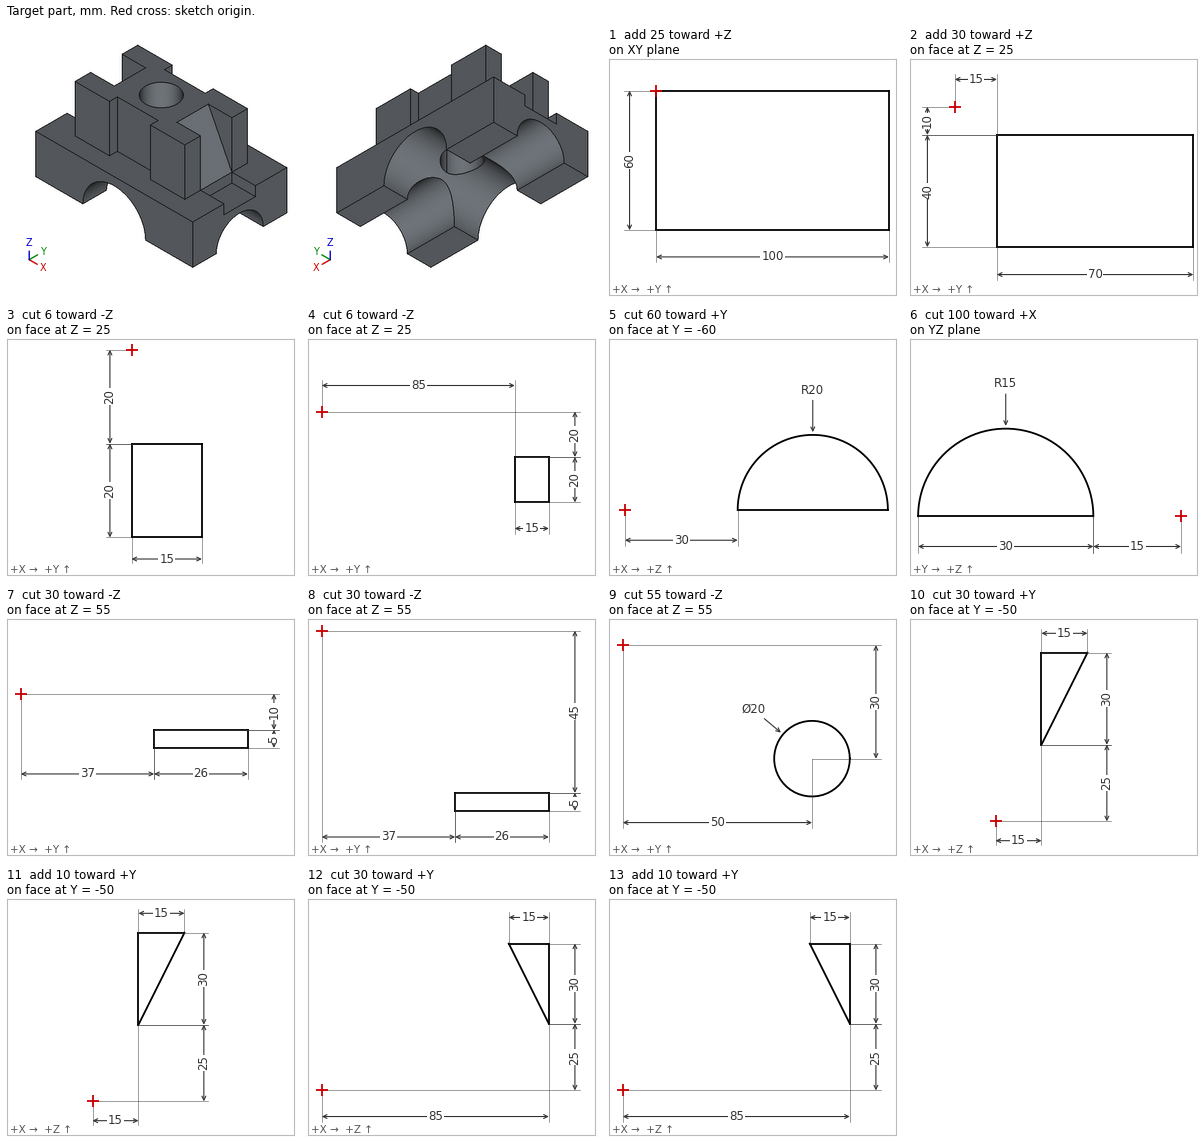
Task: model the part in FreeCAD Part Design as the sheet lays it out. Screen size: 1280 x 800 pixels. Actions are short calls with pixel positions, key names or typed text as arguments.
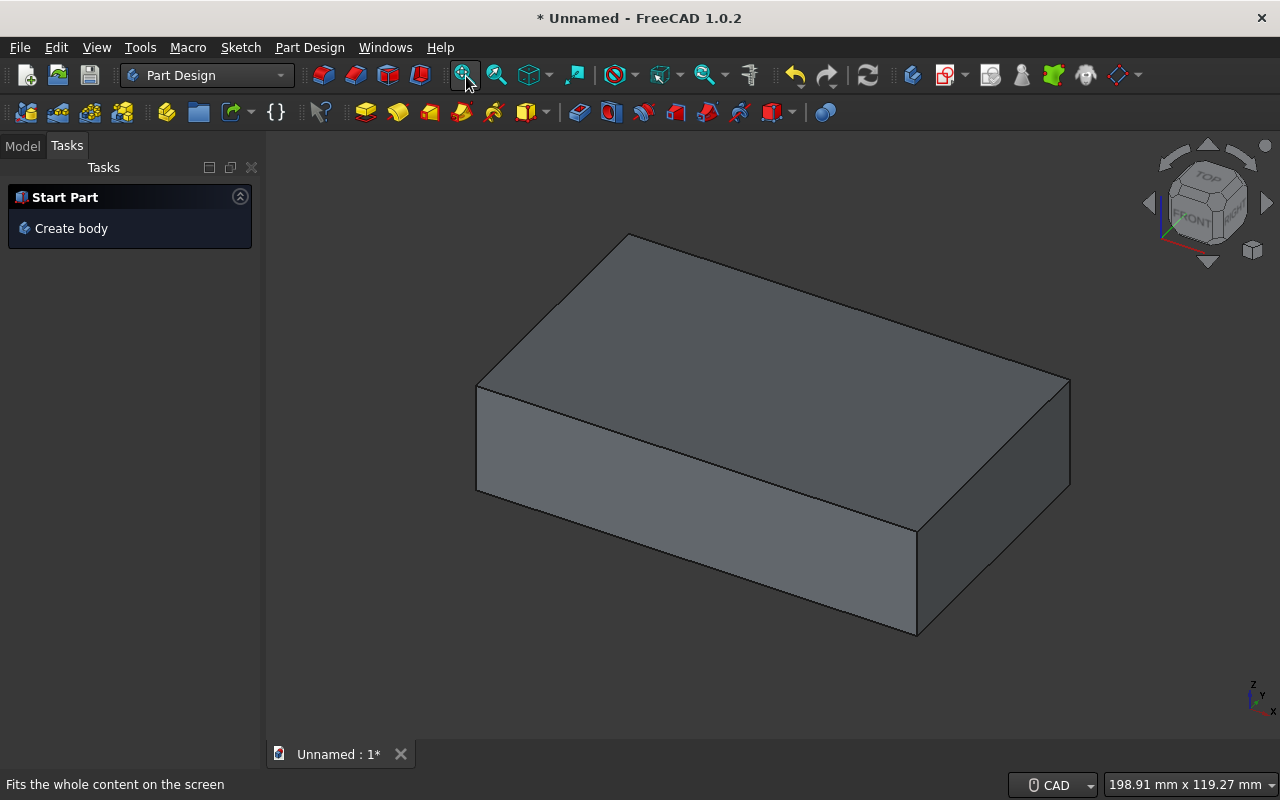
click(836, 403)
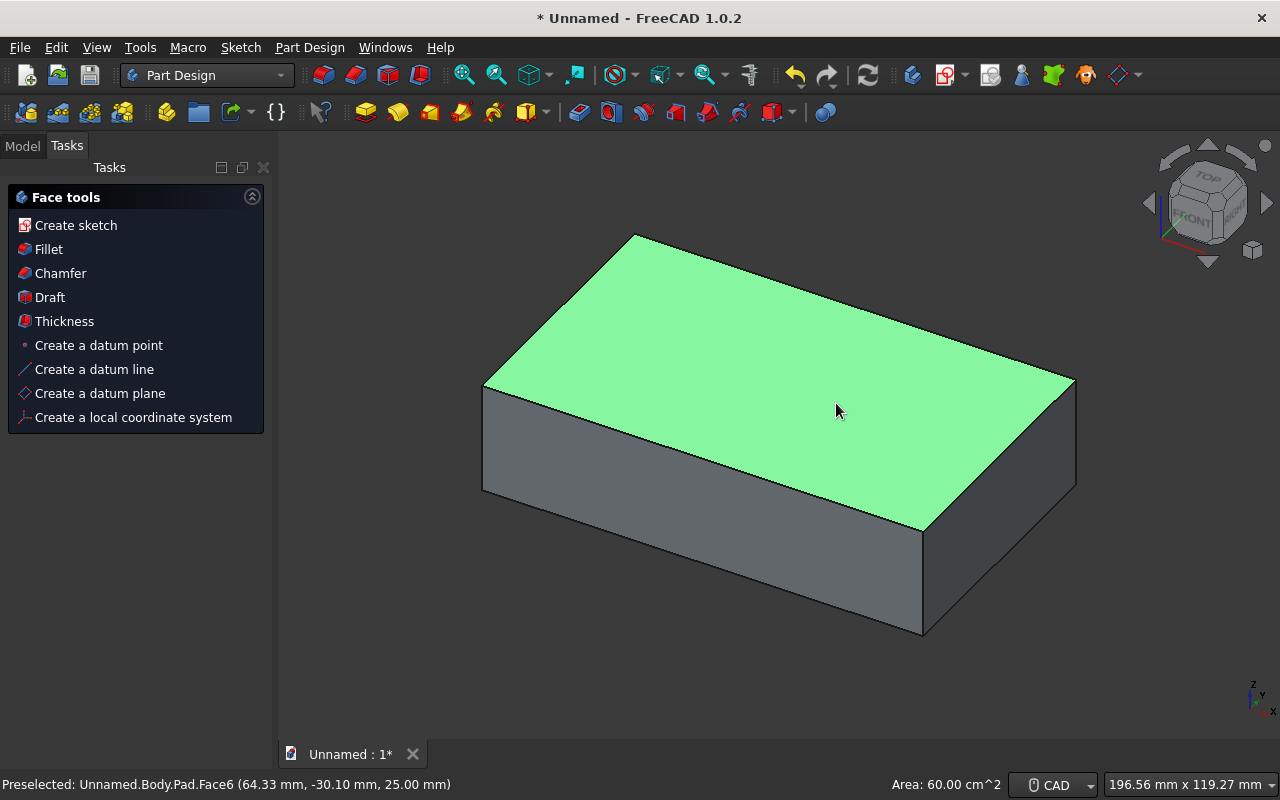
click(946, 76)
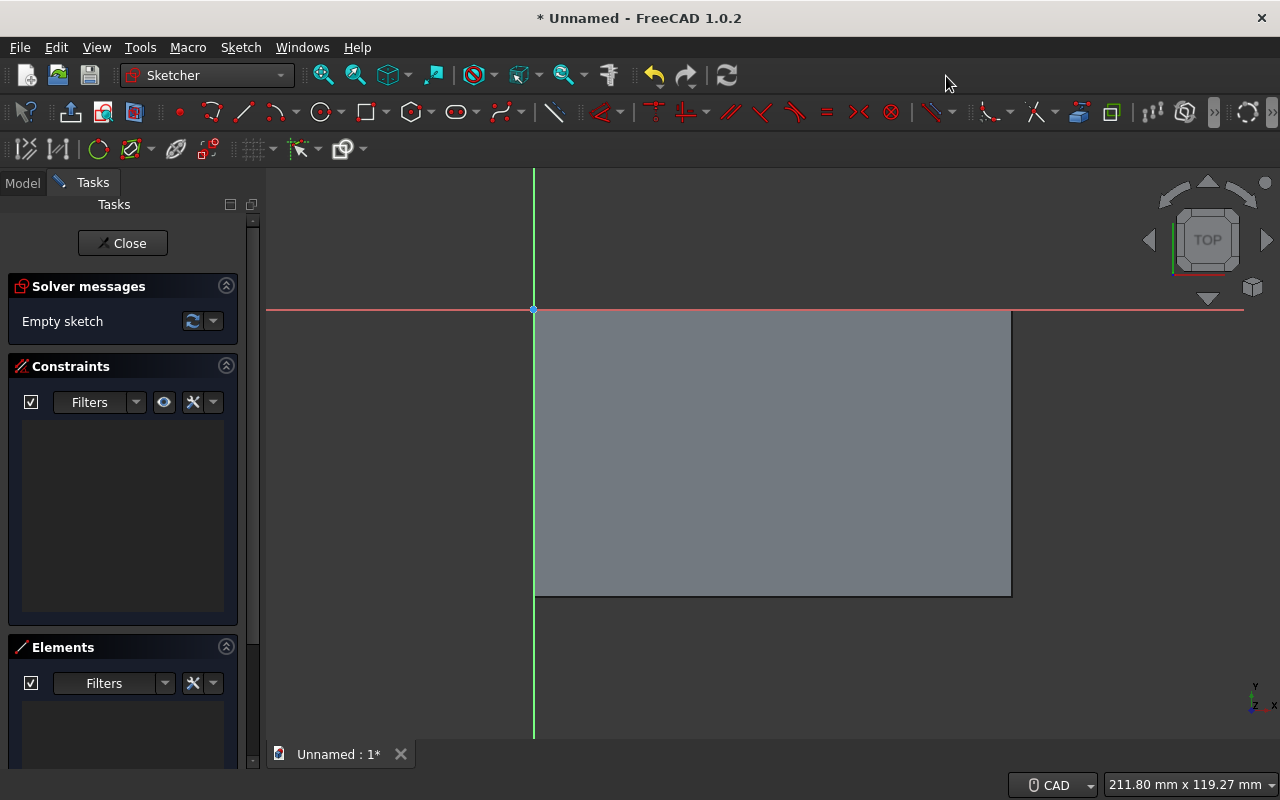
scroll(803, 381, up, 2)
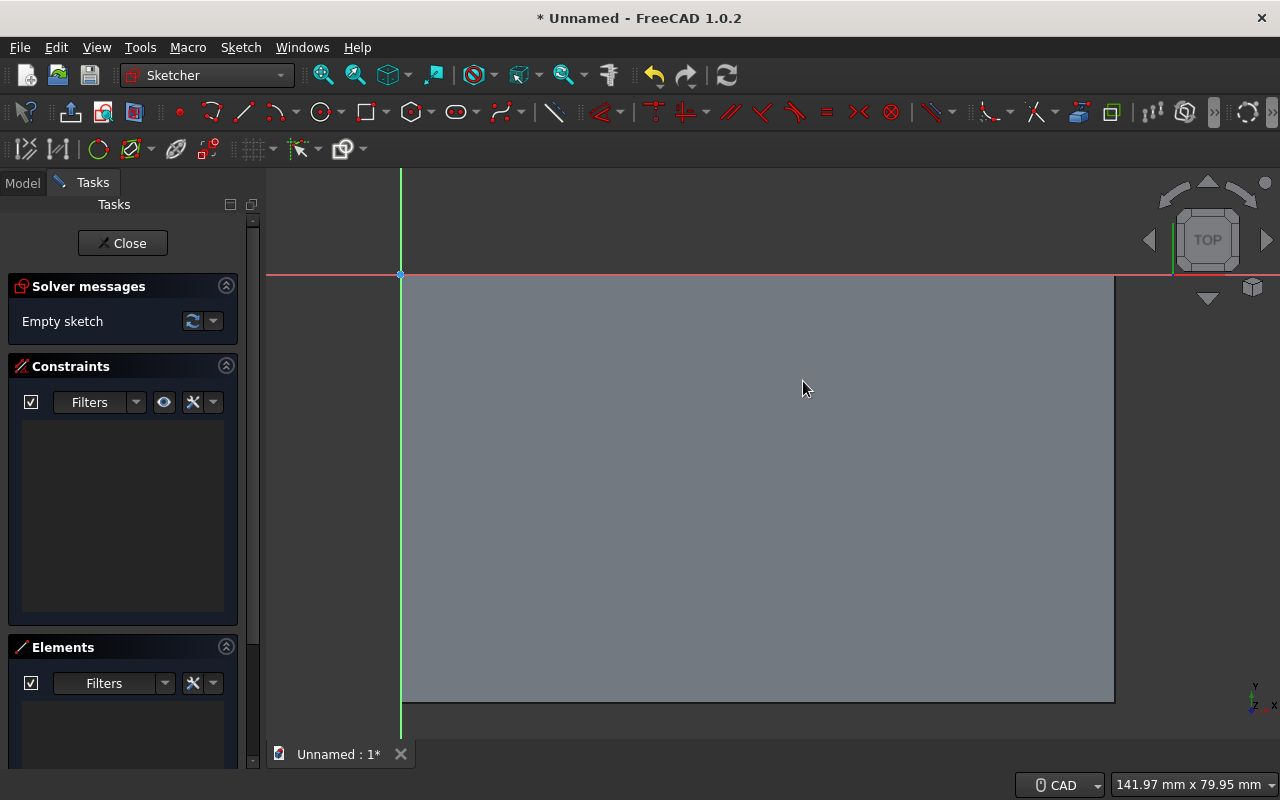
click(366, 112)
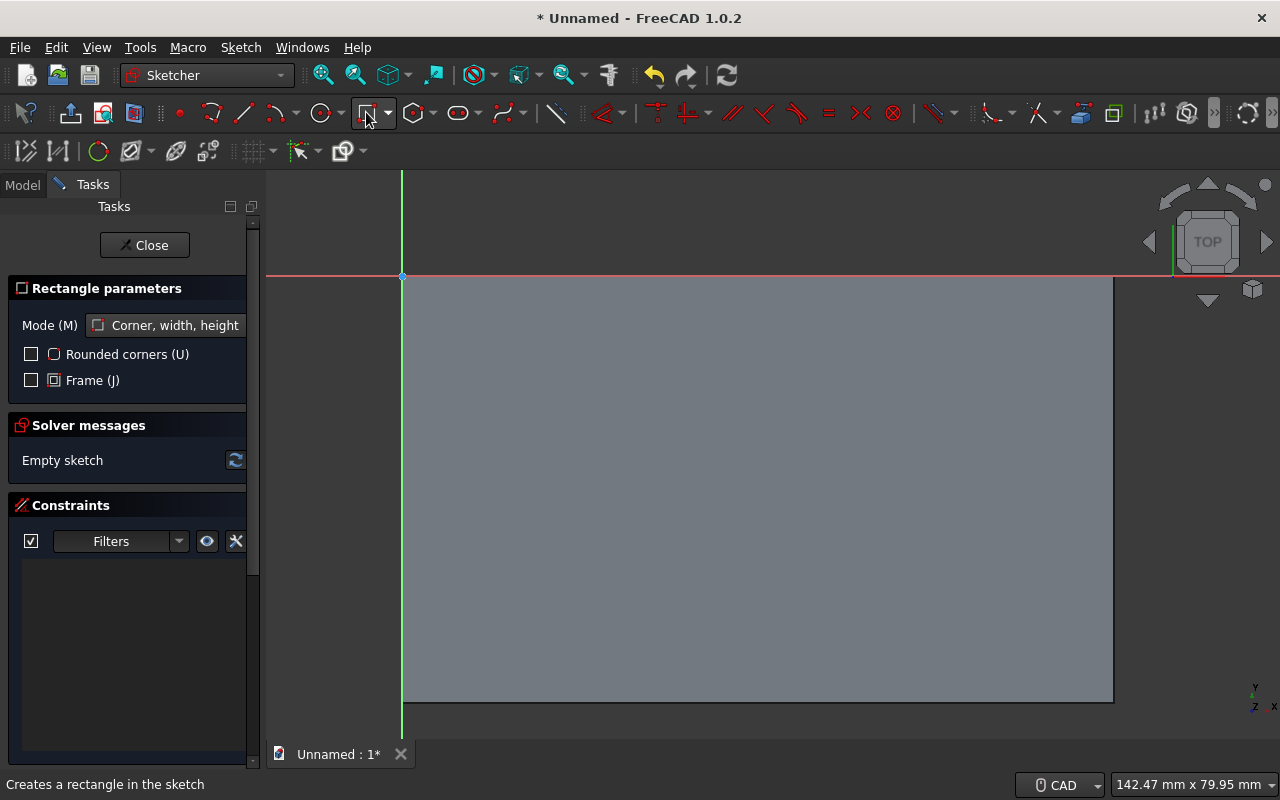
click(509, 348)
click(1007, 632)
key(Escape)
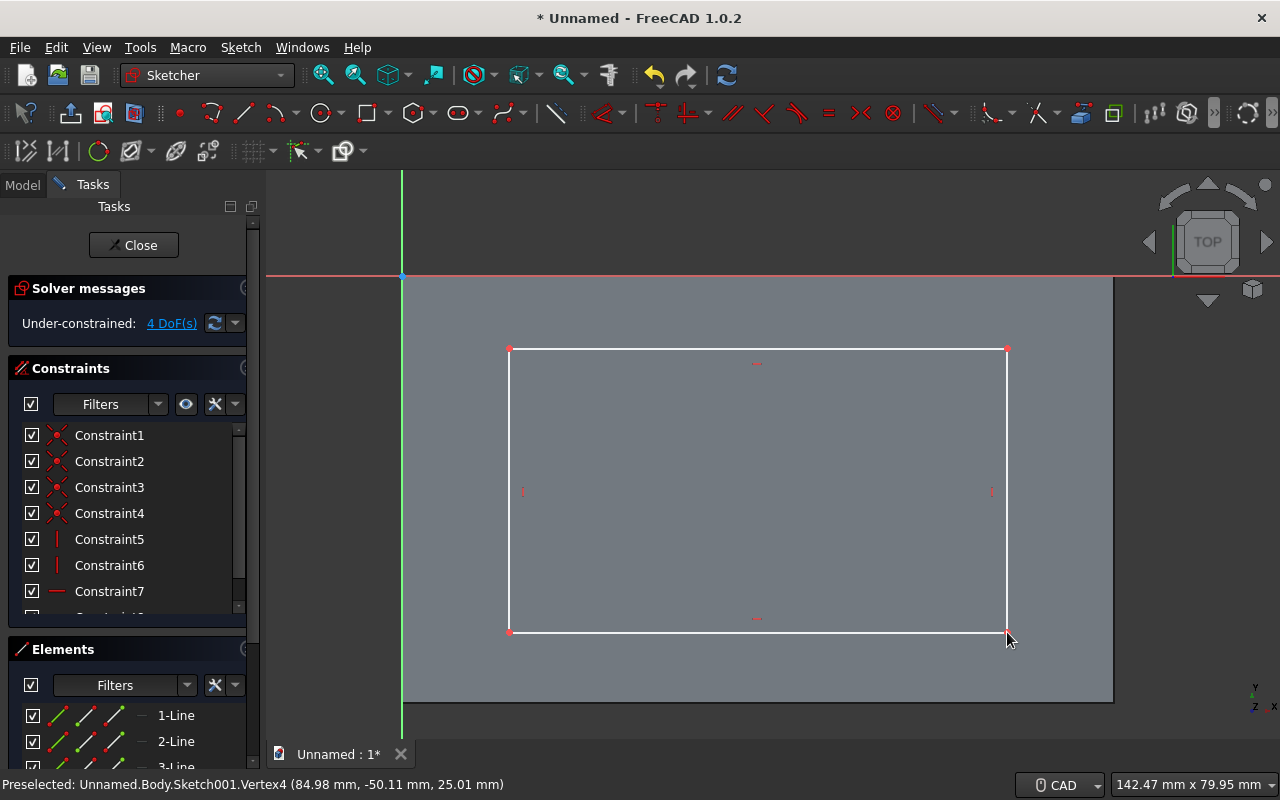
key(d)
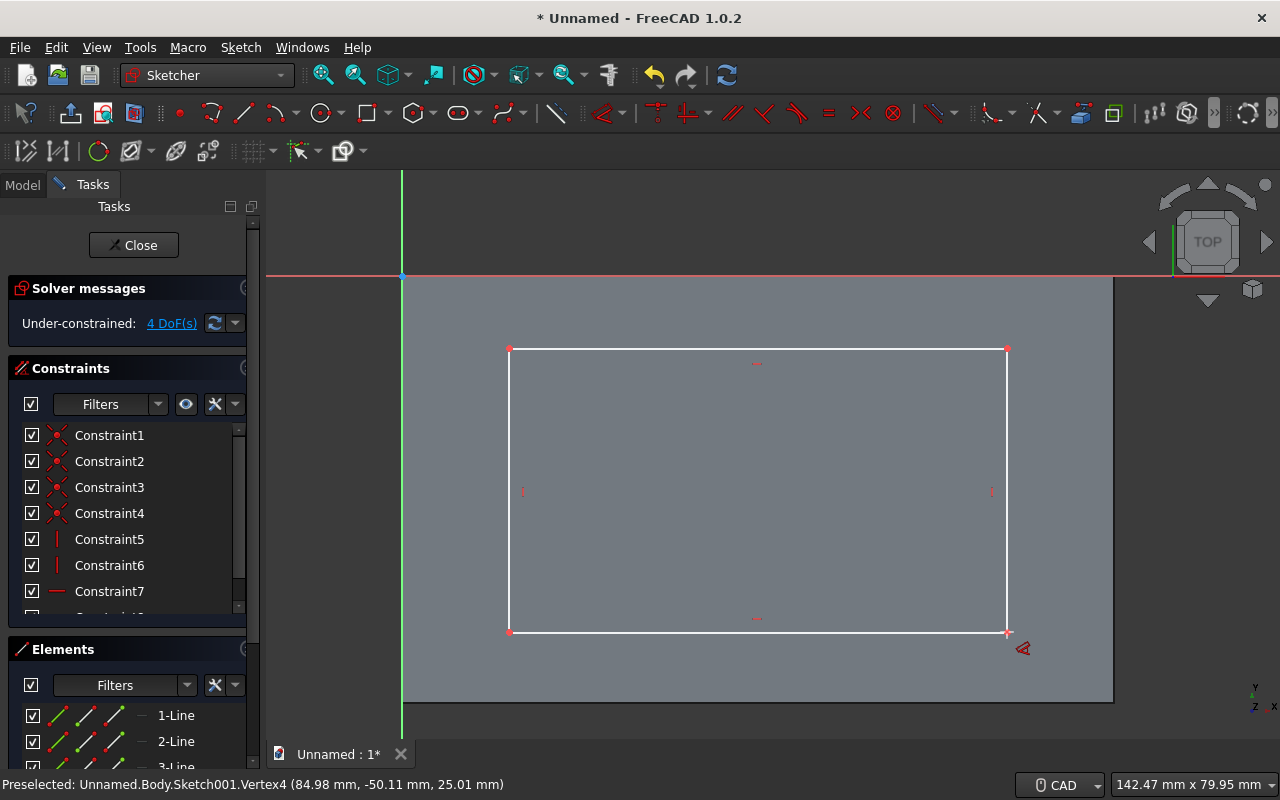
click(509, 434)
click(475, 491)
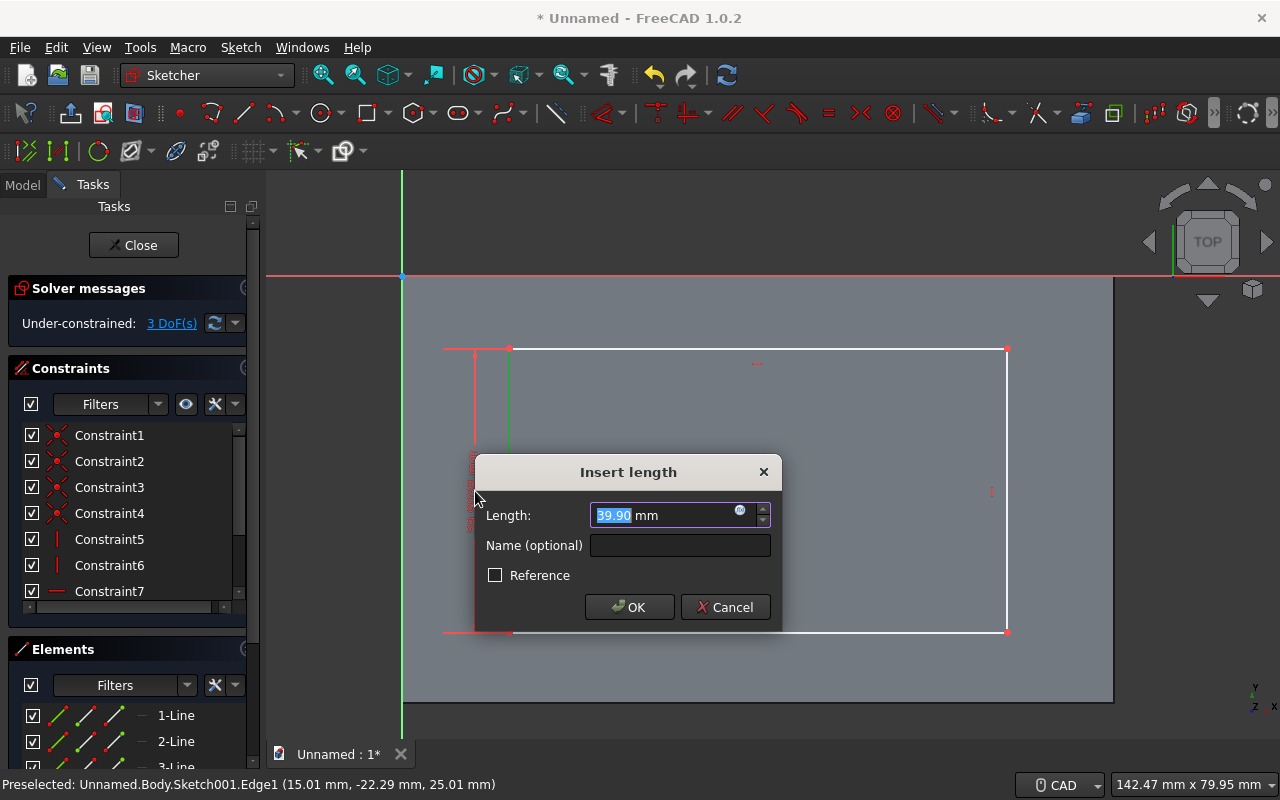
text(40)
key(Return)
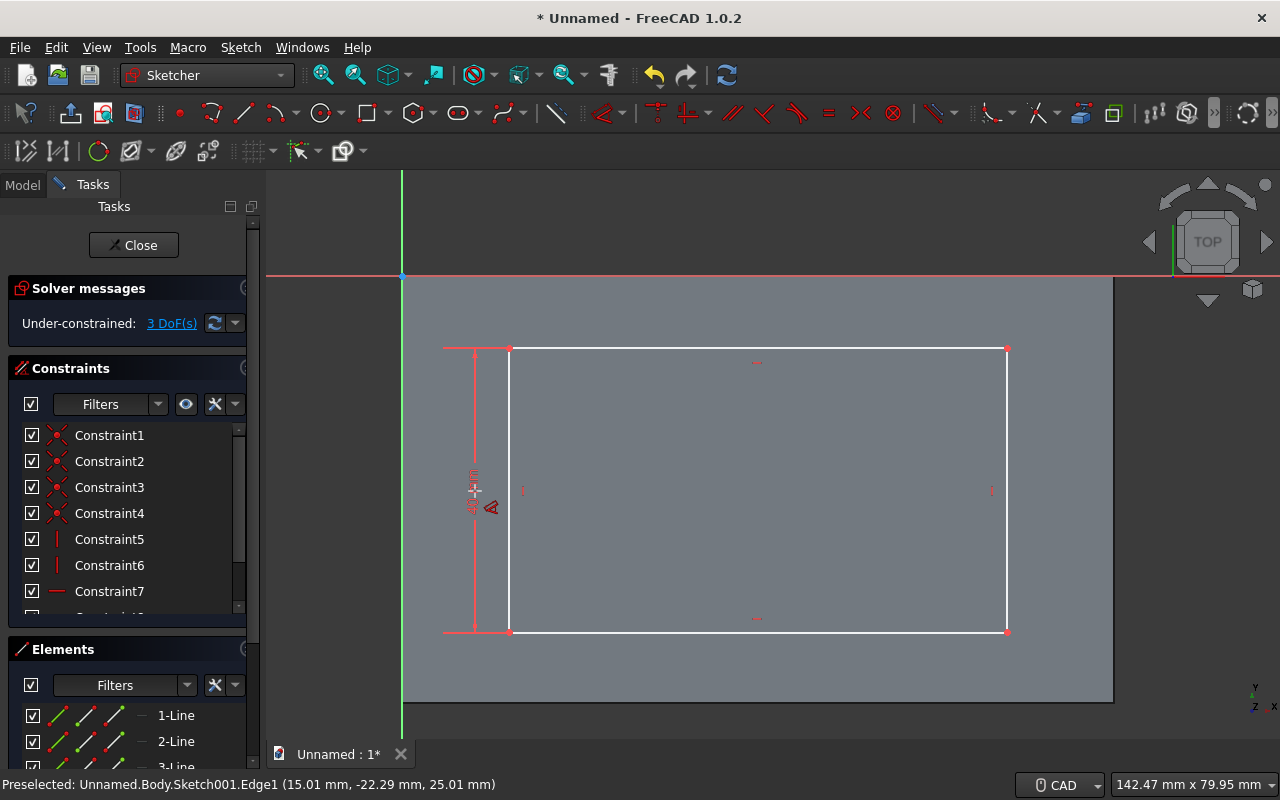
click(658, 633)
click(758, 667)